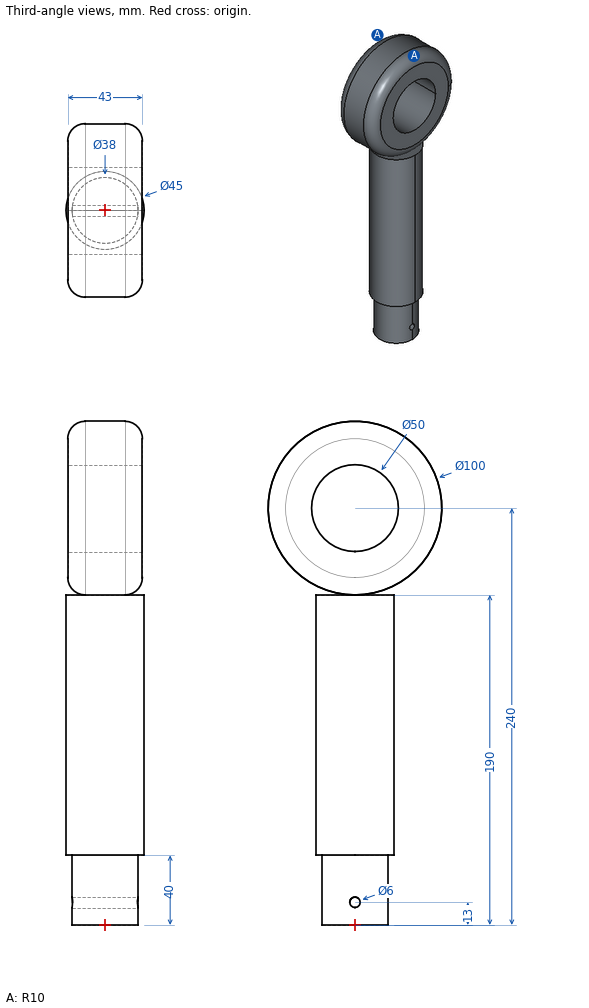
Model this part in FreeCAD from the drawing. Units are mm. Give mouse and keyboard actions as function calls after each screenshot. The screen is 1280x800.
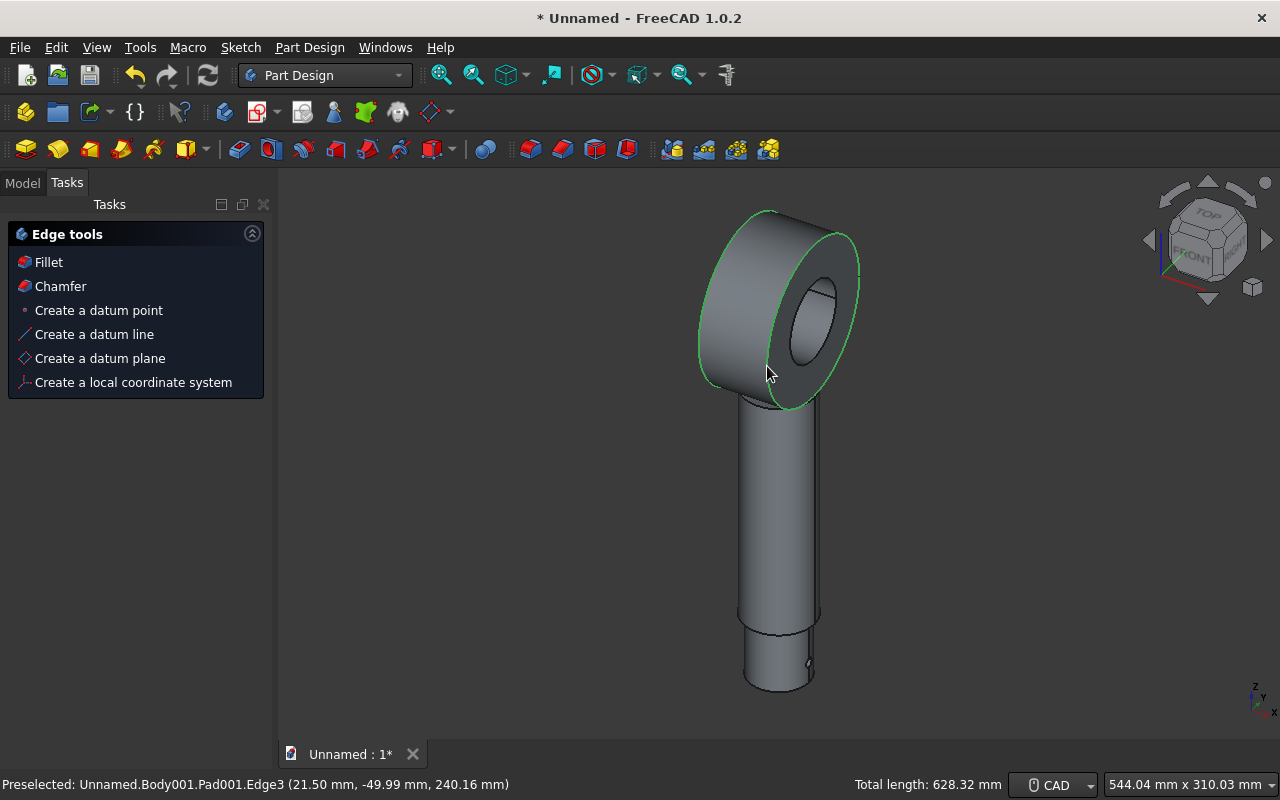
click(532, 150)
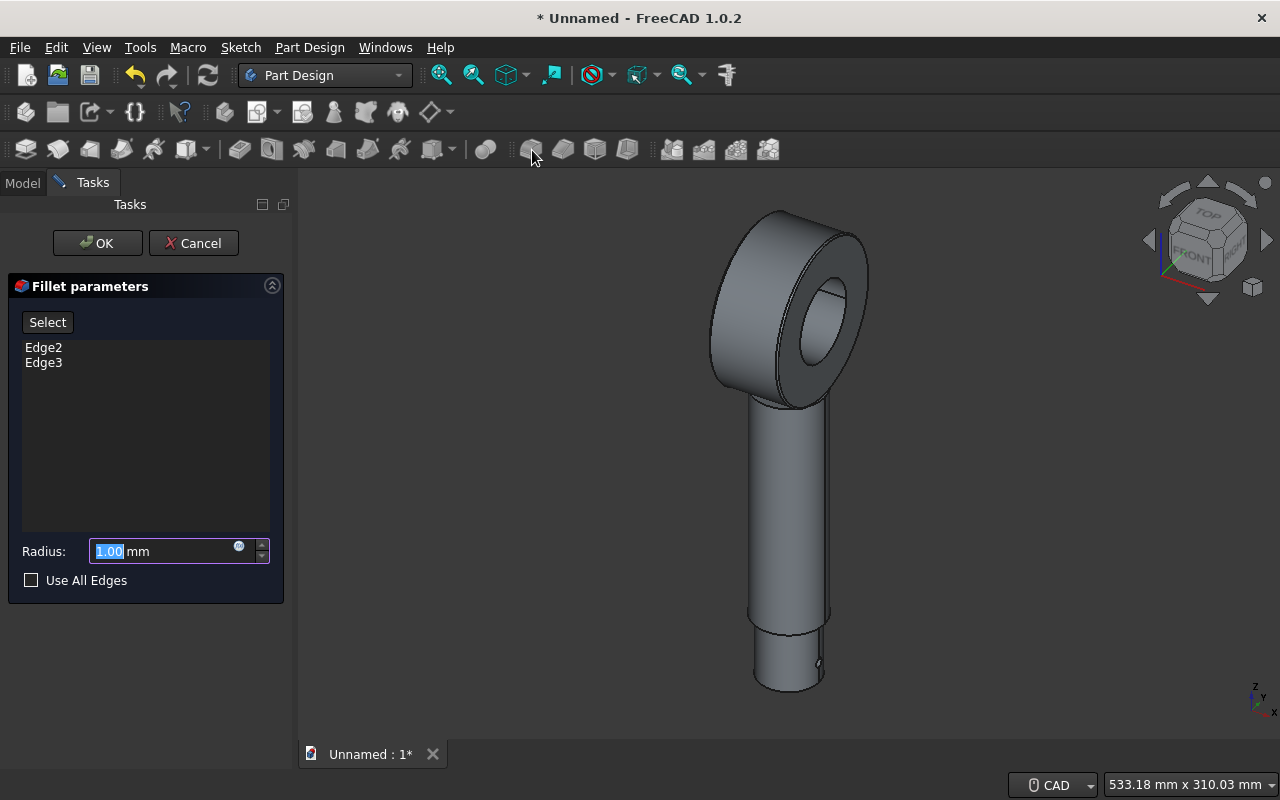
text(10)
key(Tab)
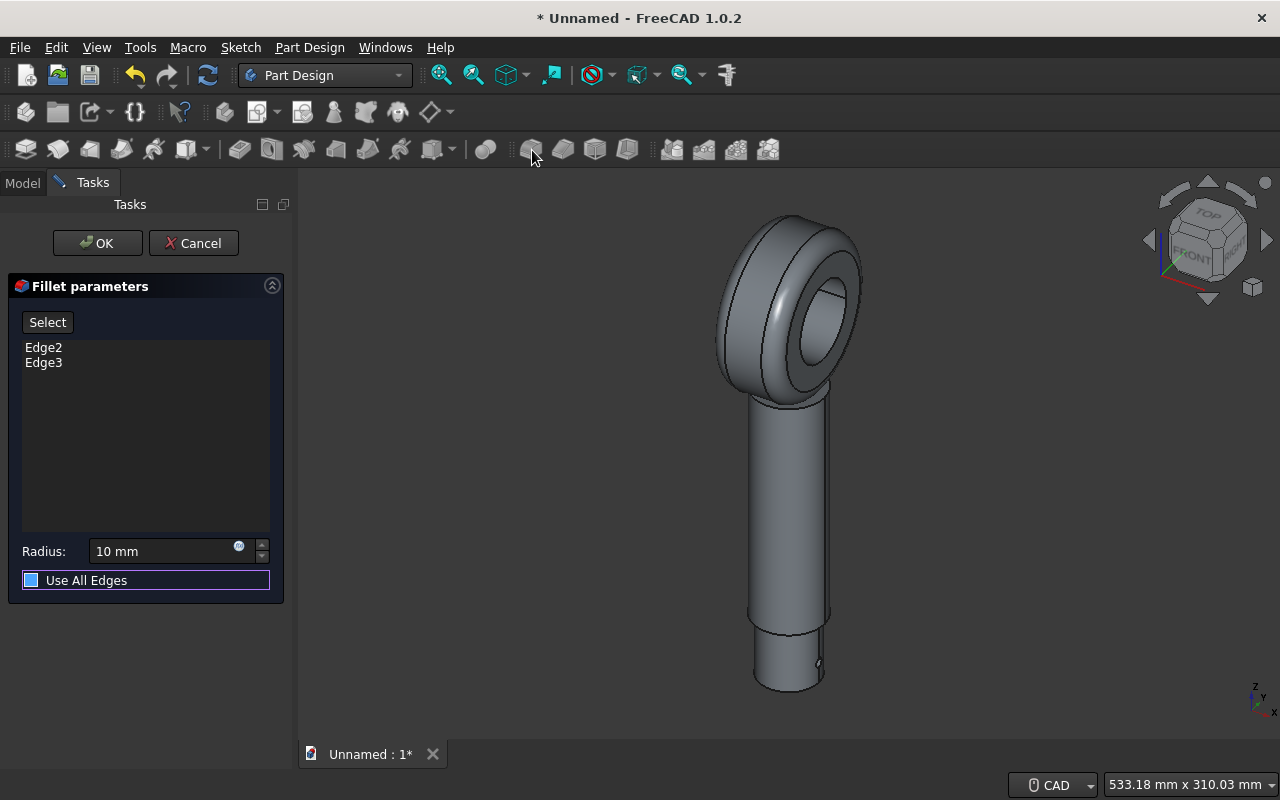
click(98, 243)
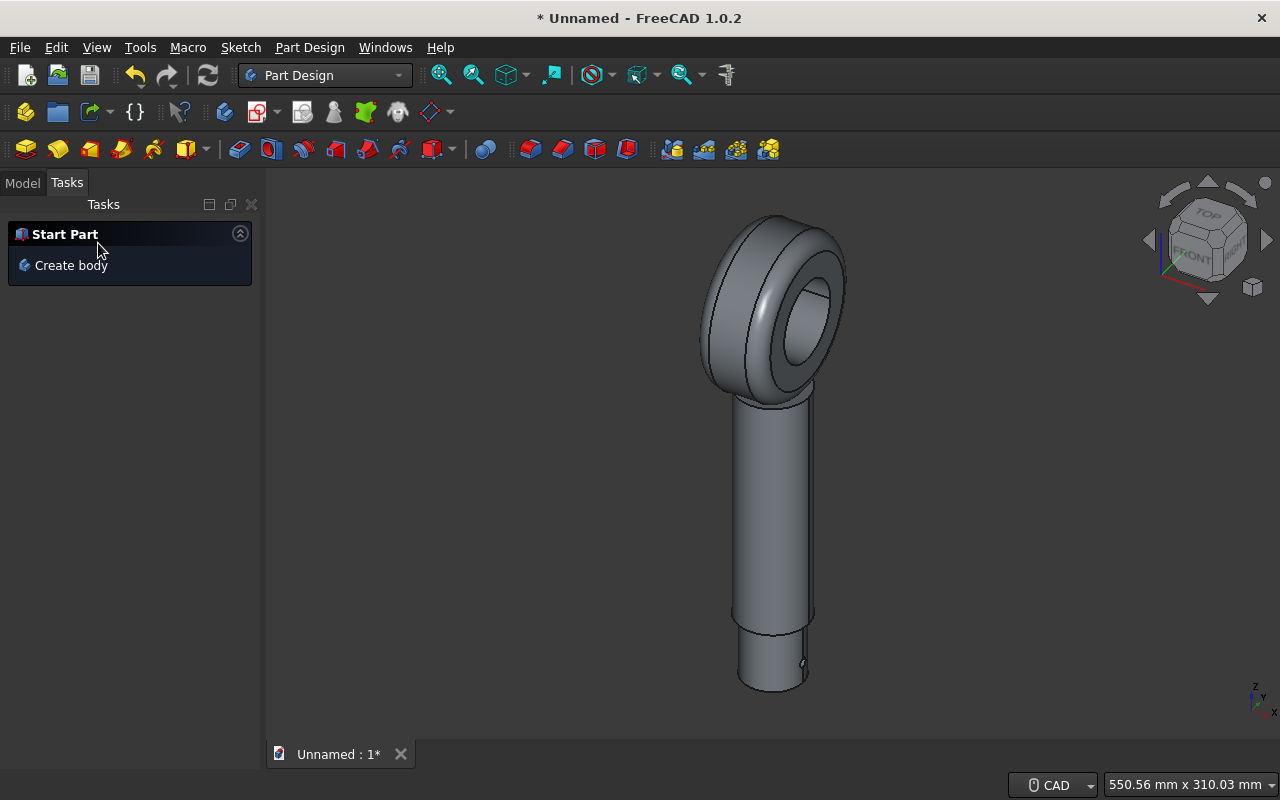
key(0)